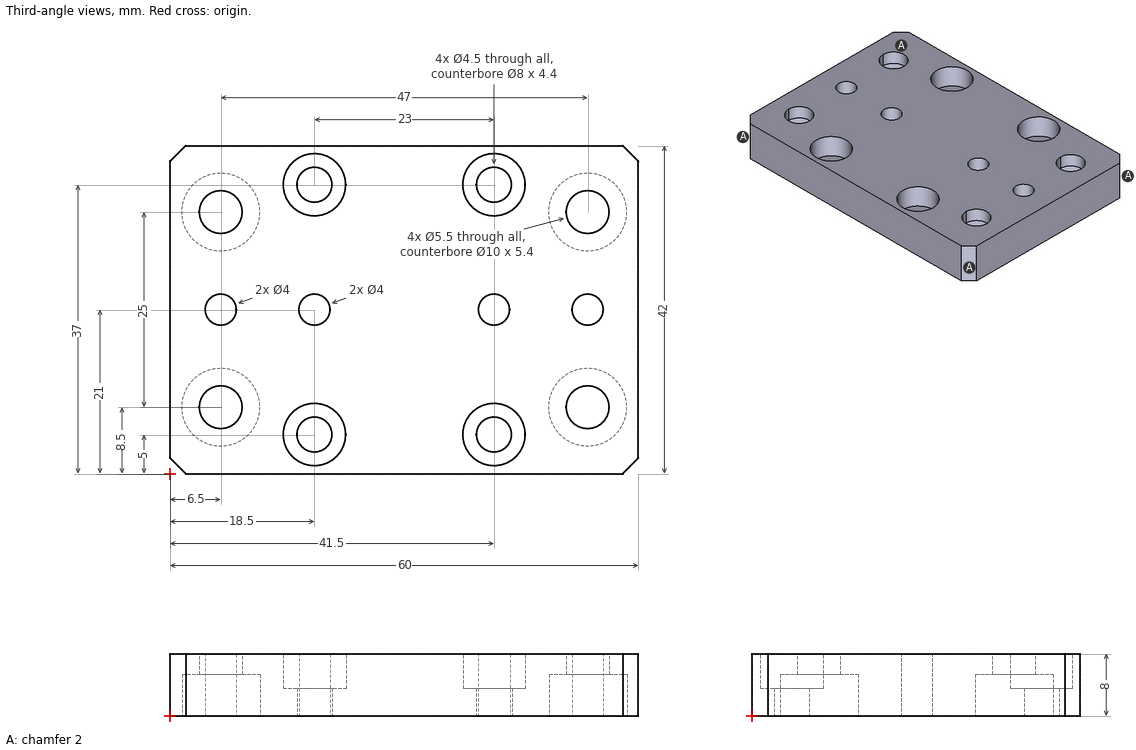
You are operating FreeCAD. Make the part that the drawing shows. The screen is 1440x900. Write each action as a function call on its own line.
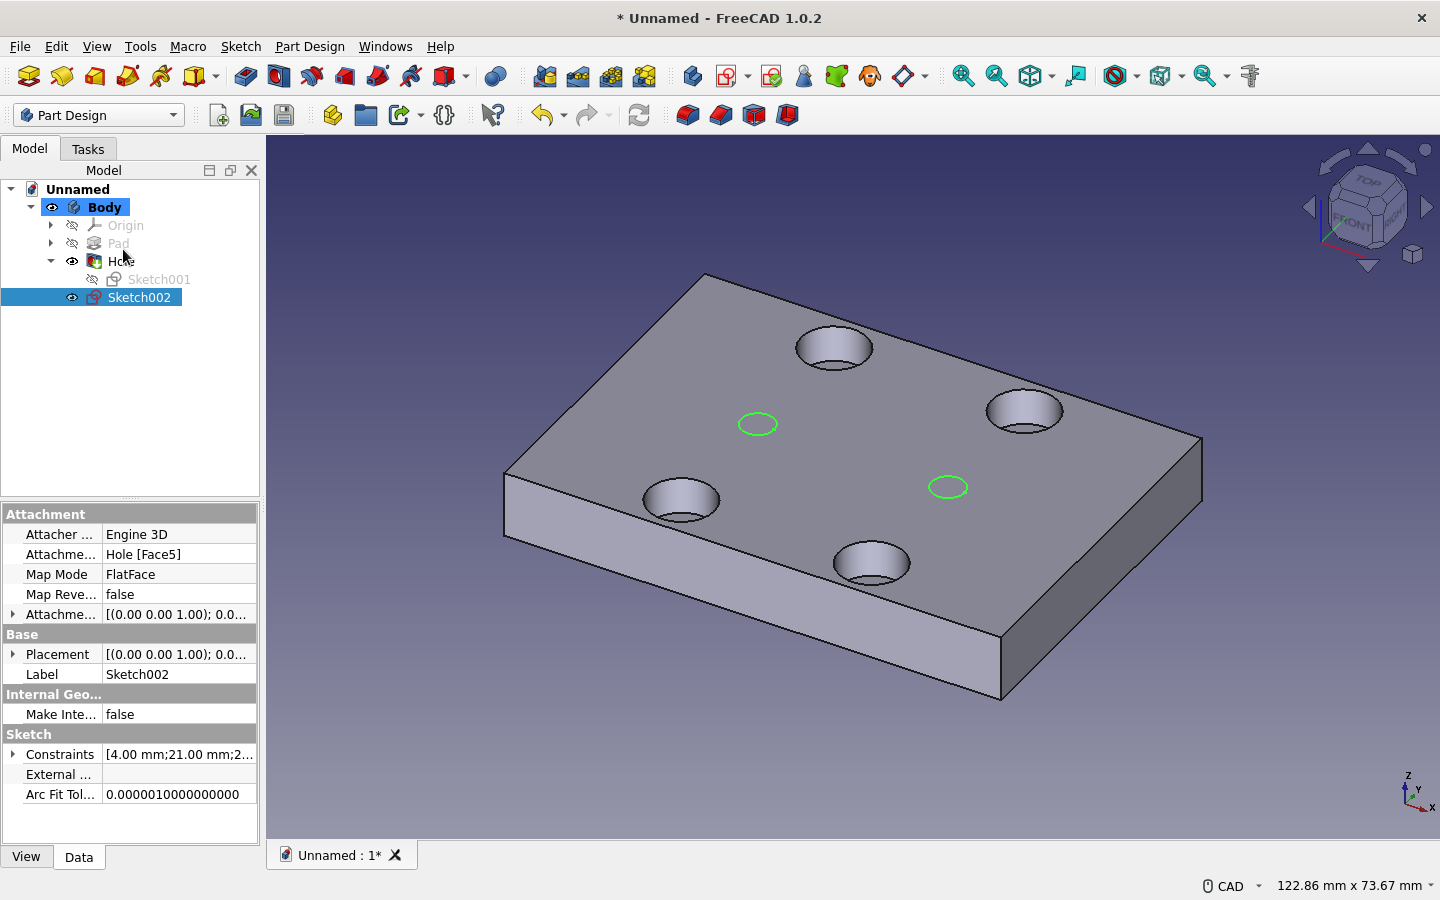
click(246, 76)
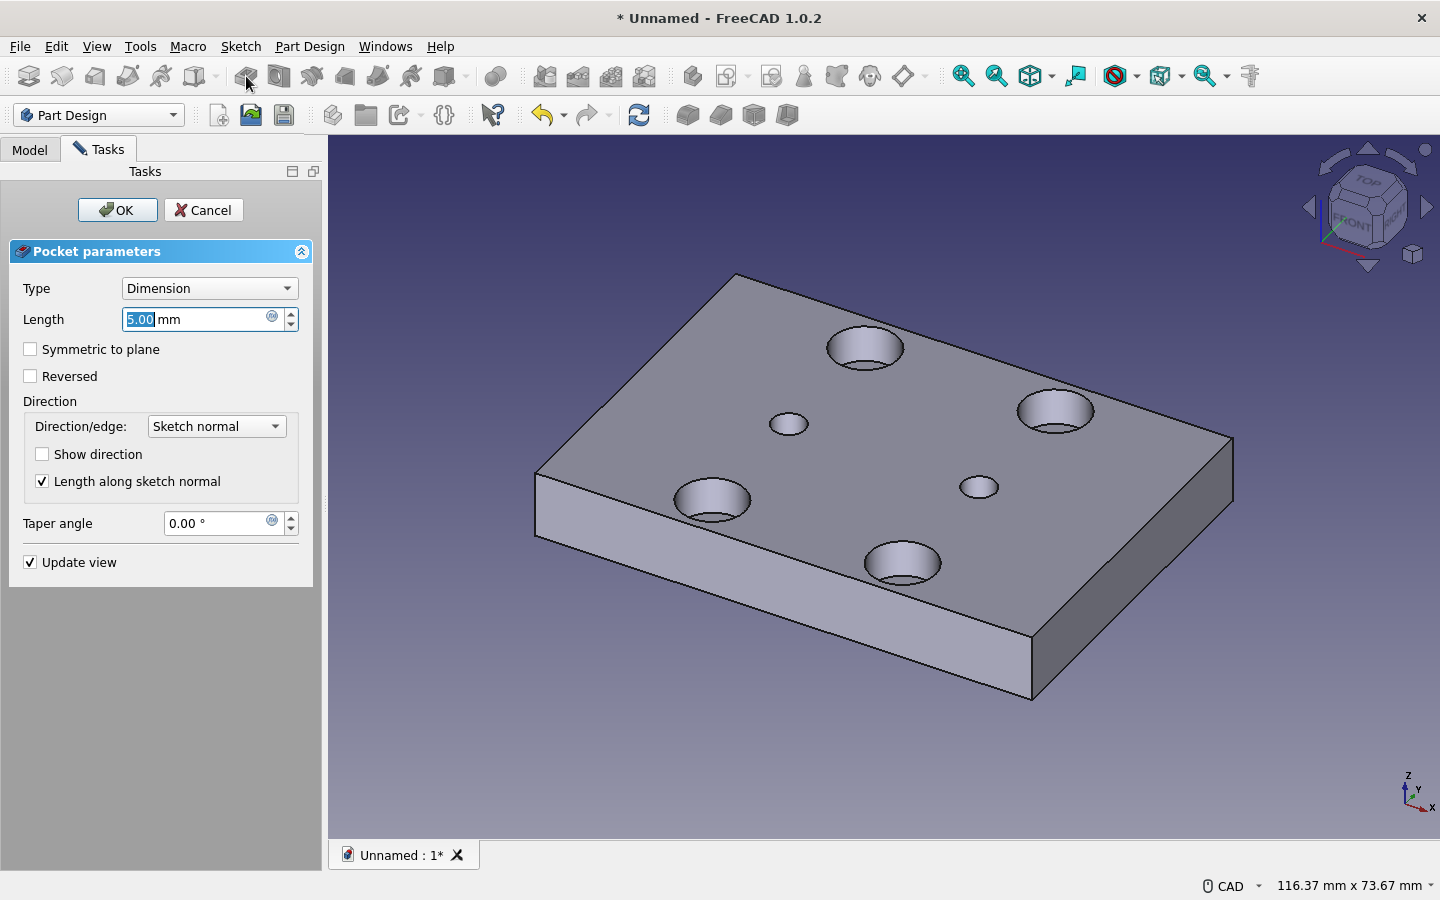
click(210, 288)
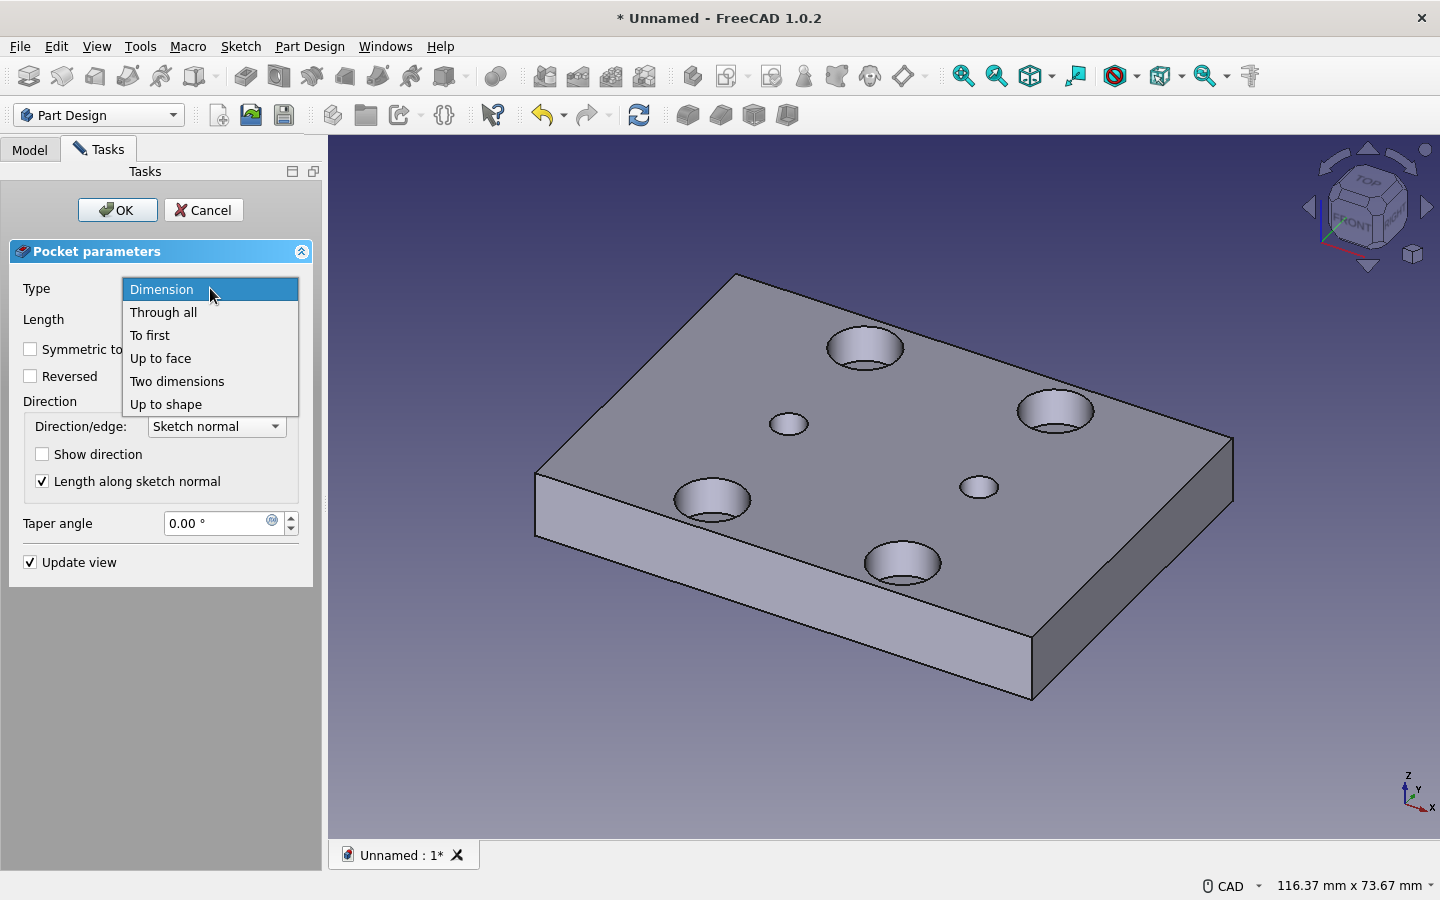
click(208, 312)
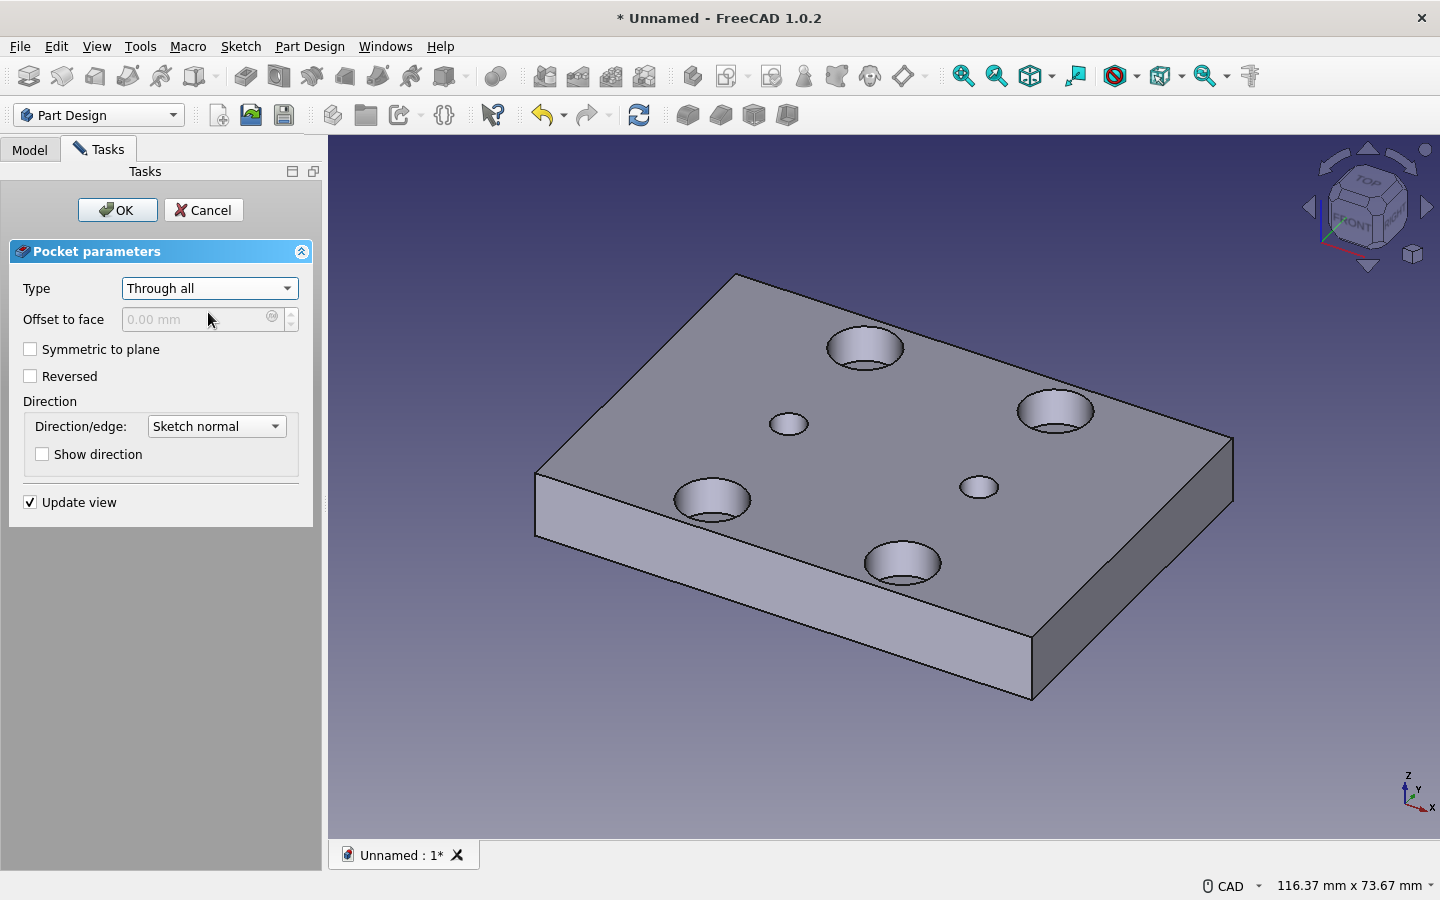
click(118, 210)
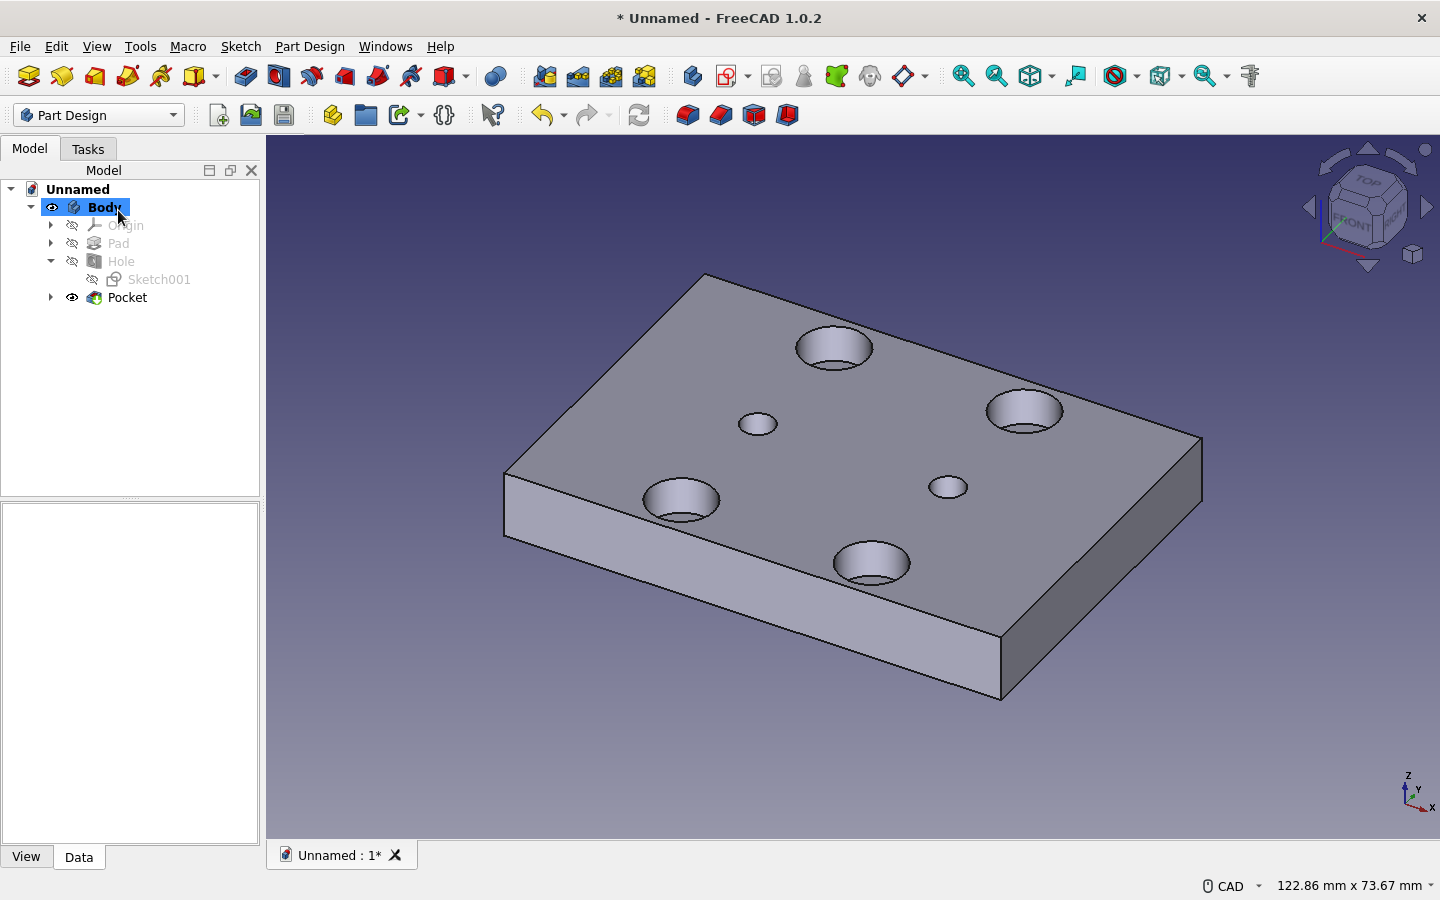
click(726, 76)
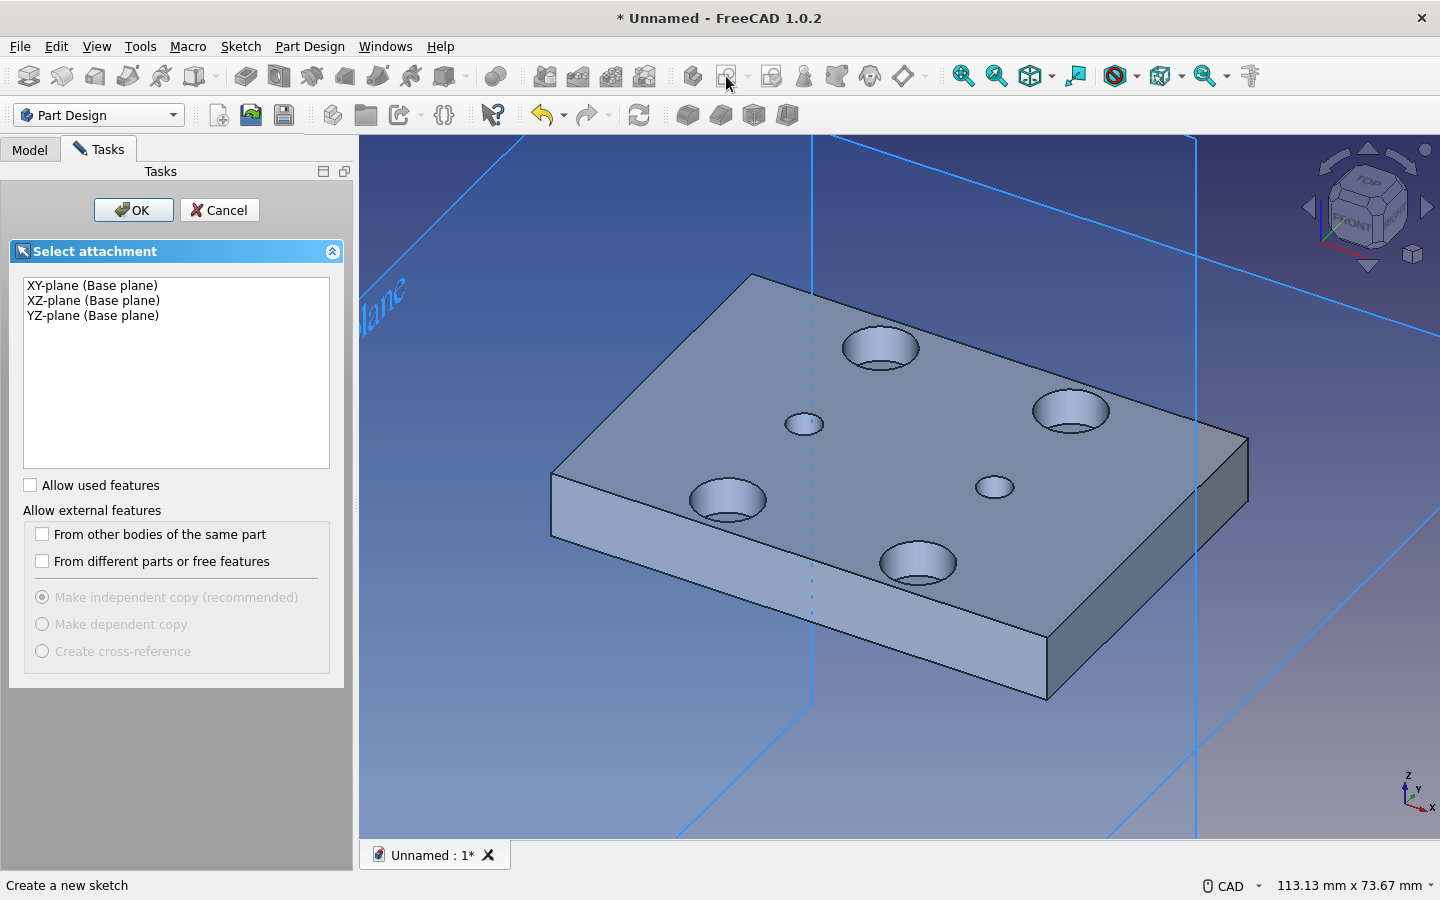
click(84, 286)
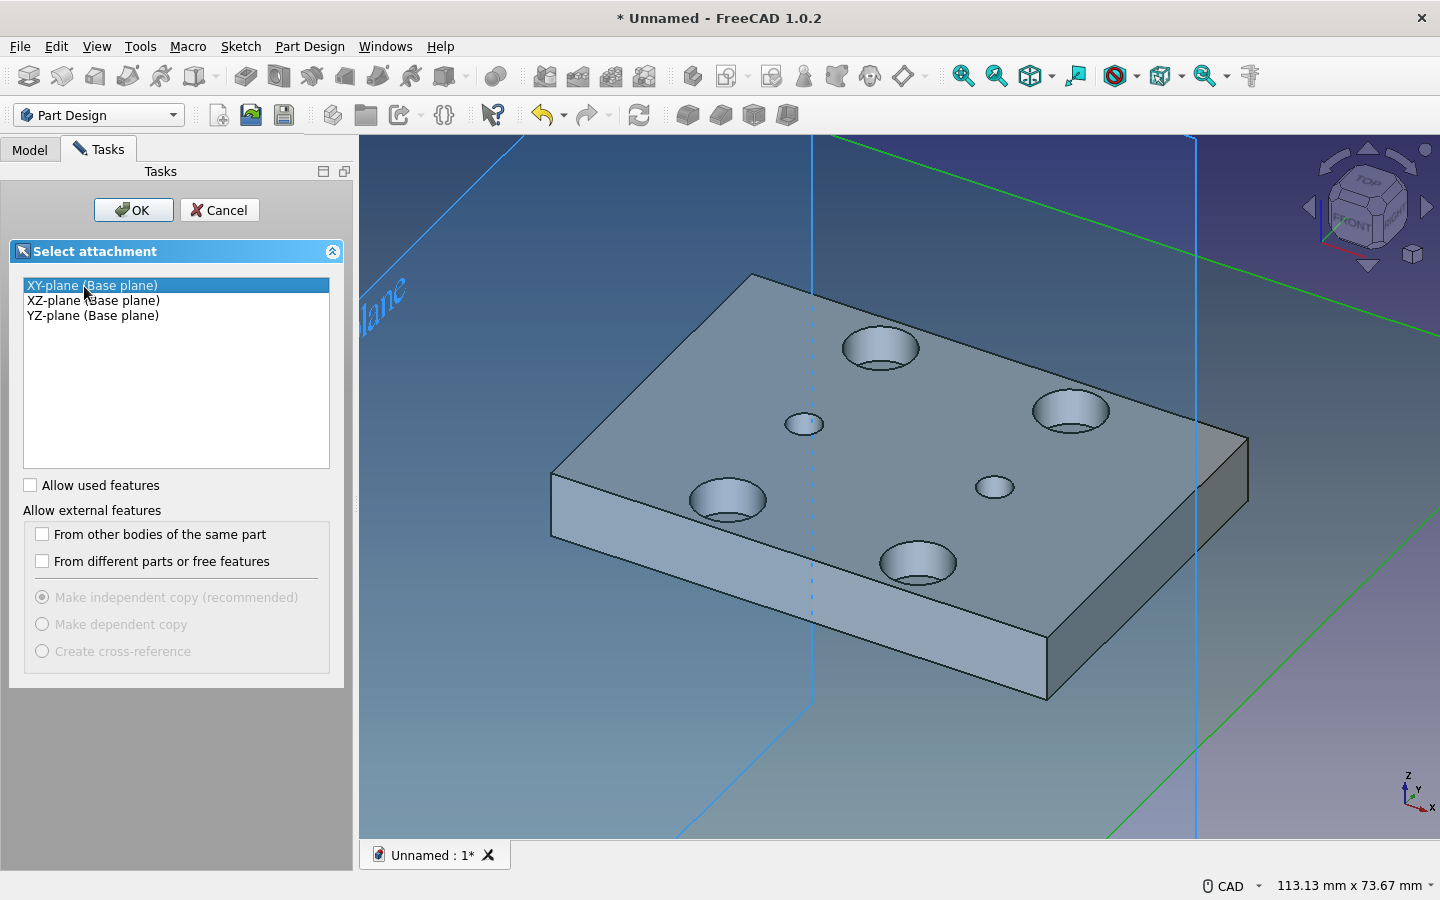
click(134, 210)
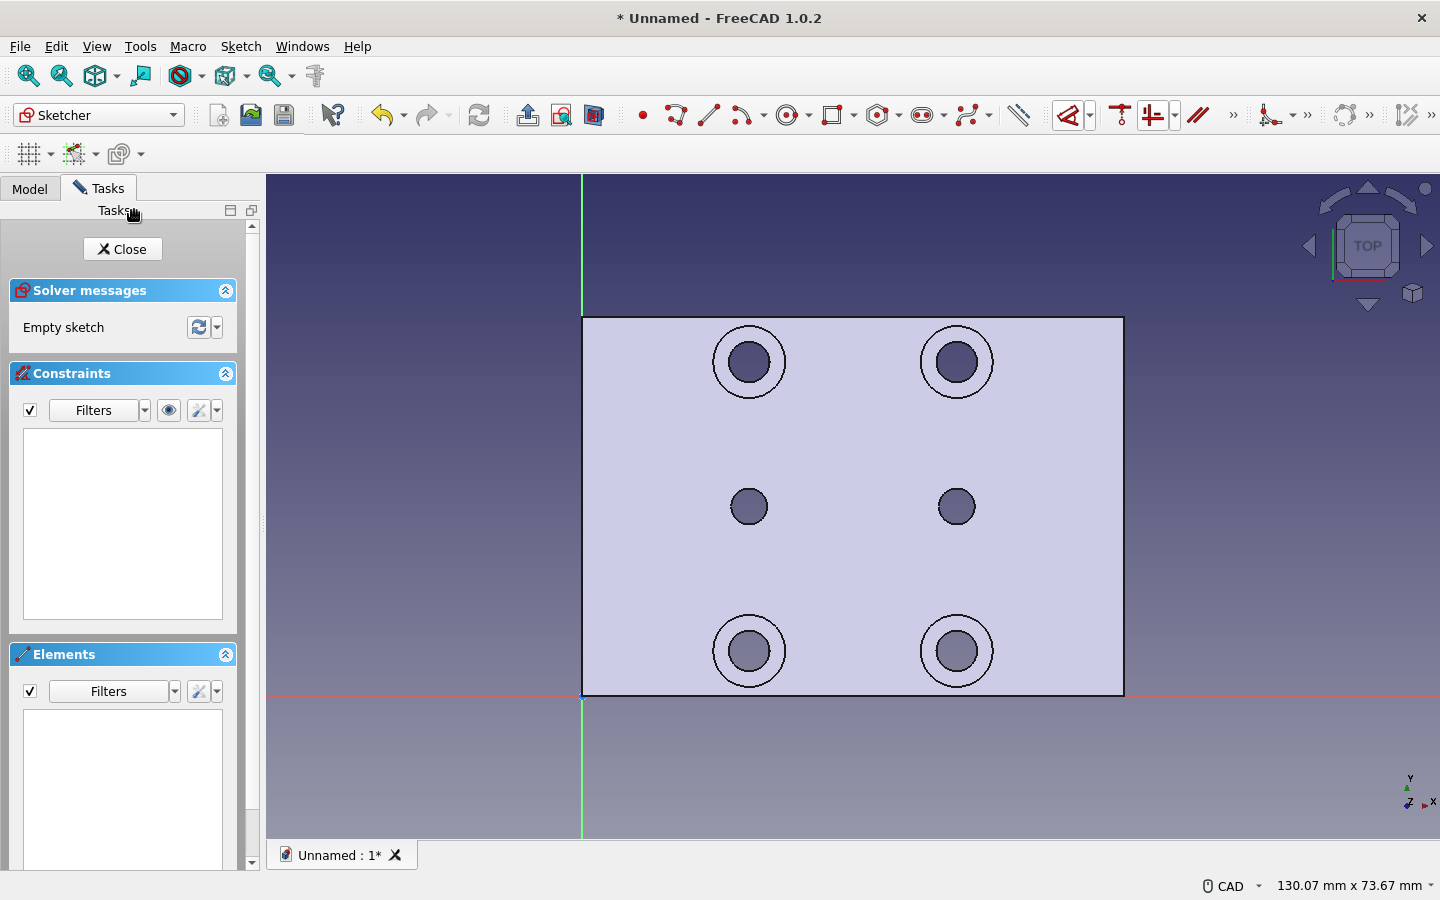
click(594, 116)